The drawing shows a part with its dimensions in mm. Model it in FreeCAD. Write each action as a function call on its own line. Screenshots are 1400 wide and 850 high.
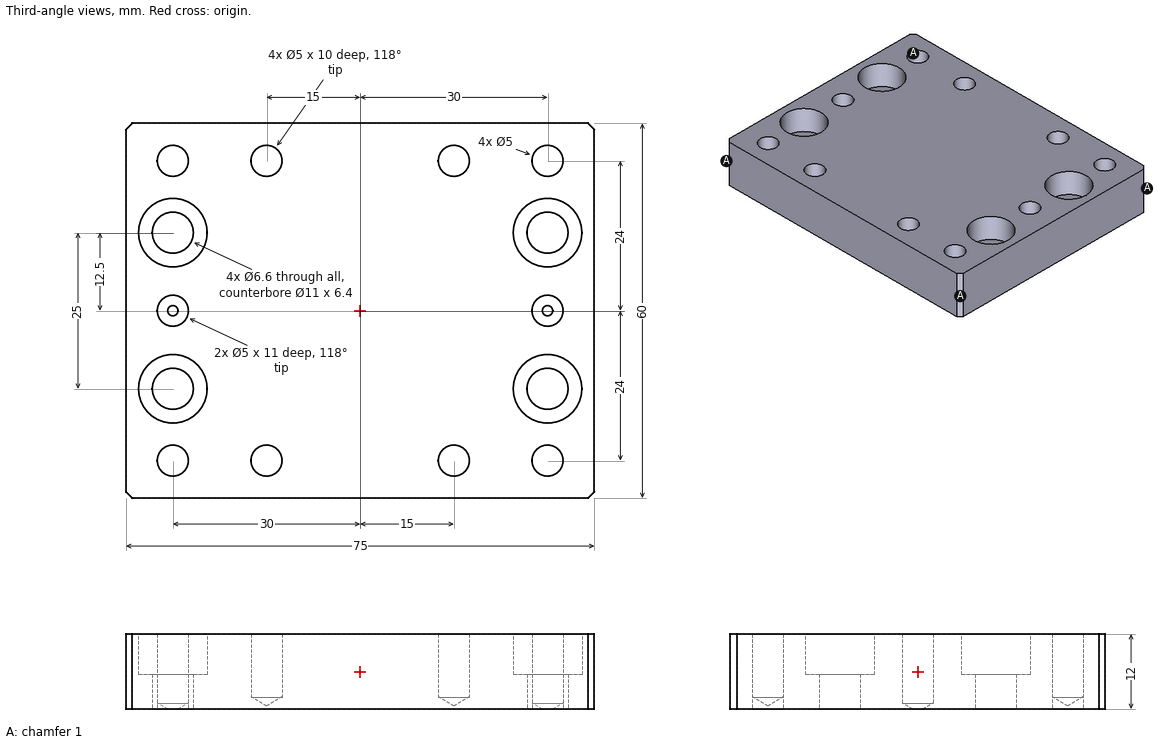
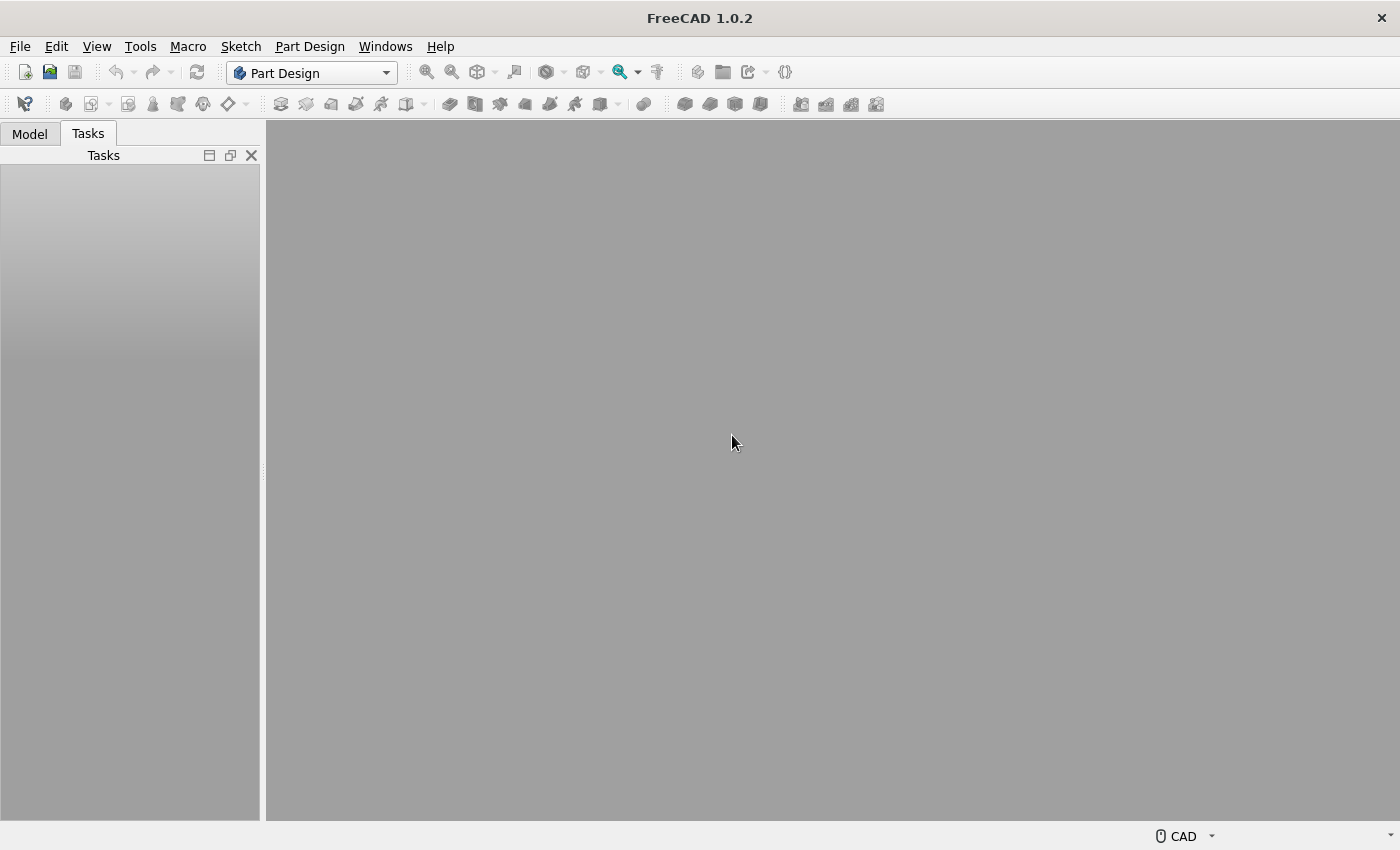
key(ctrl+n)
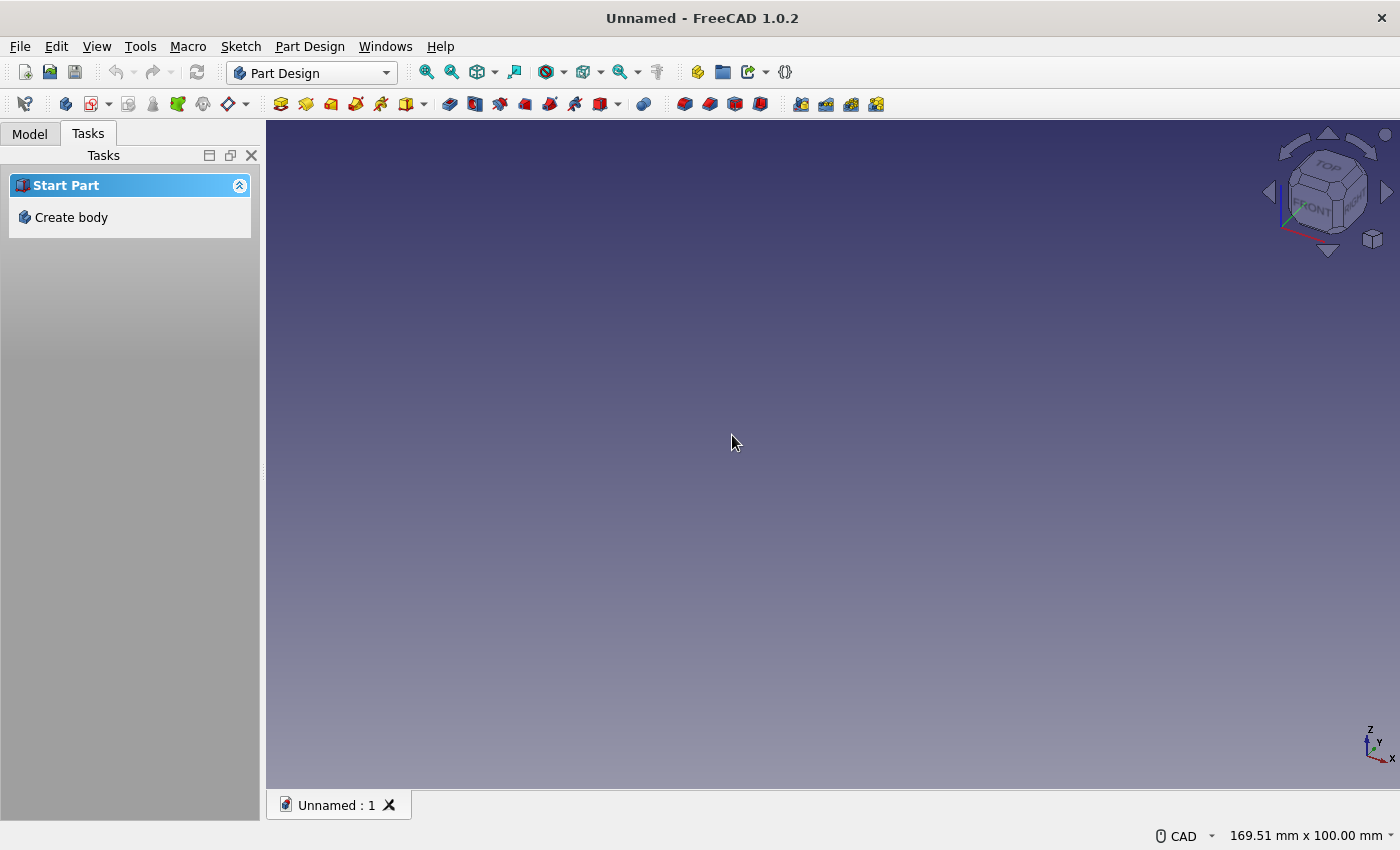
click(90, 104)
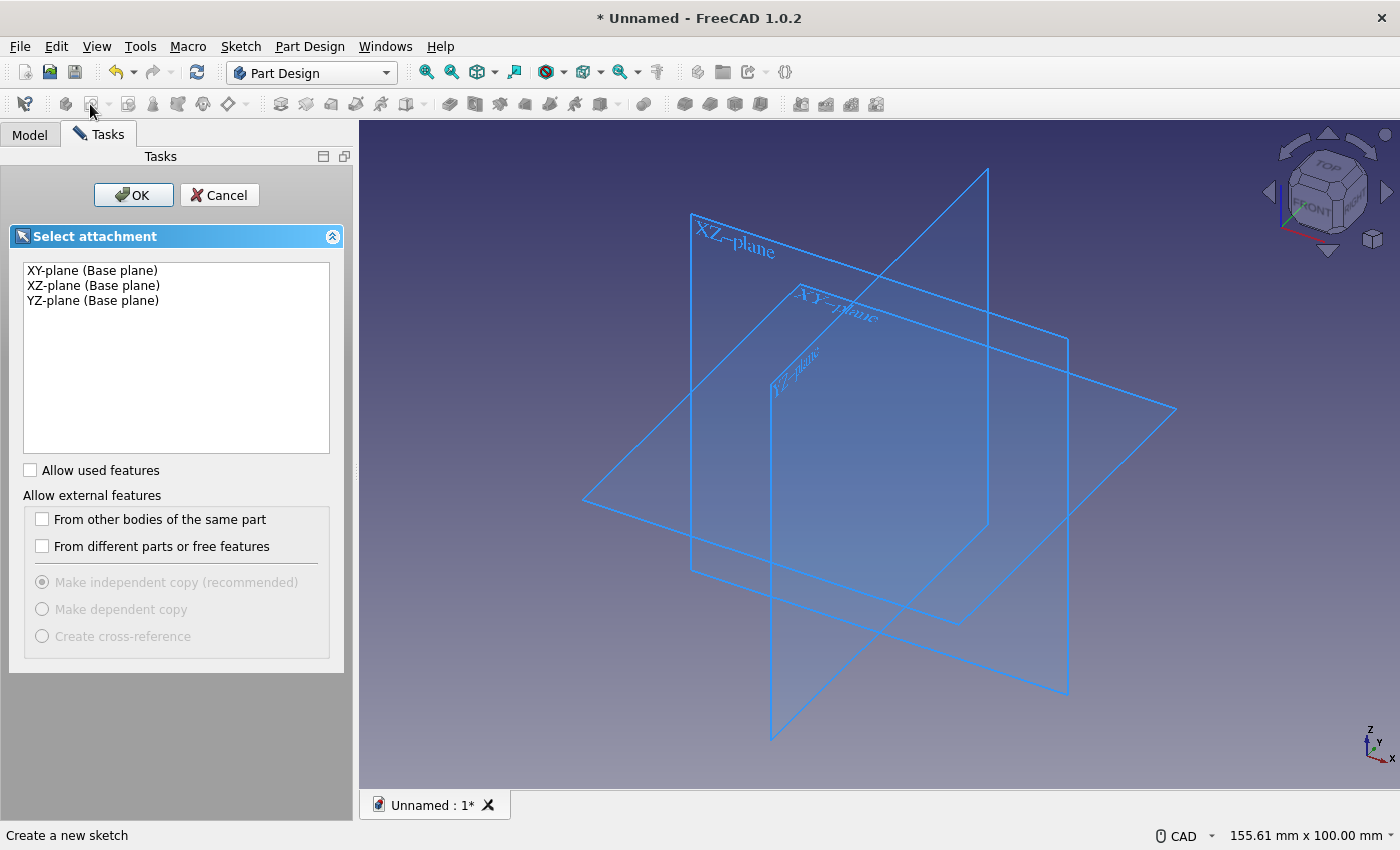
click(84, 270)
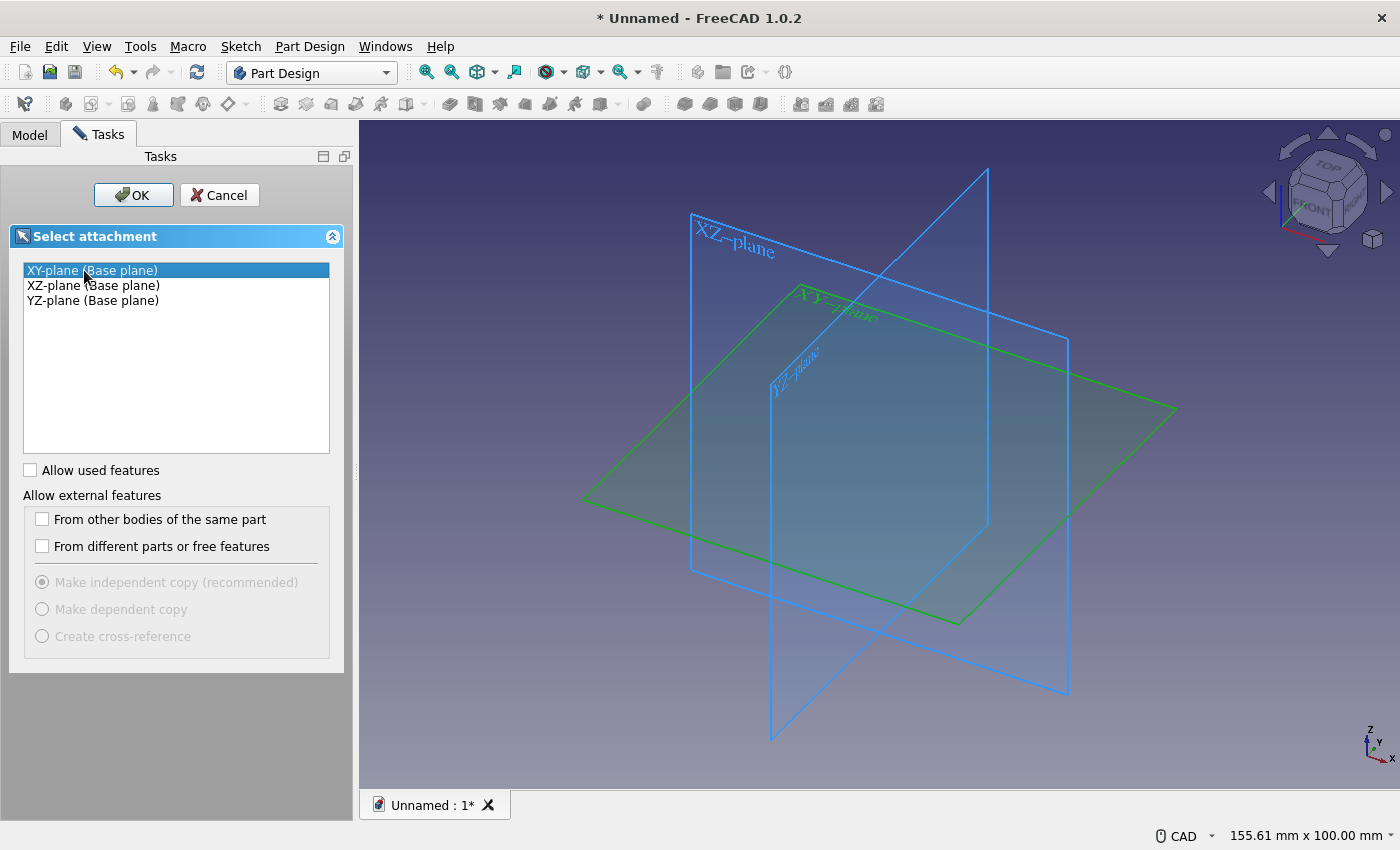
click(134, 195)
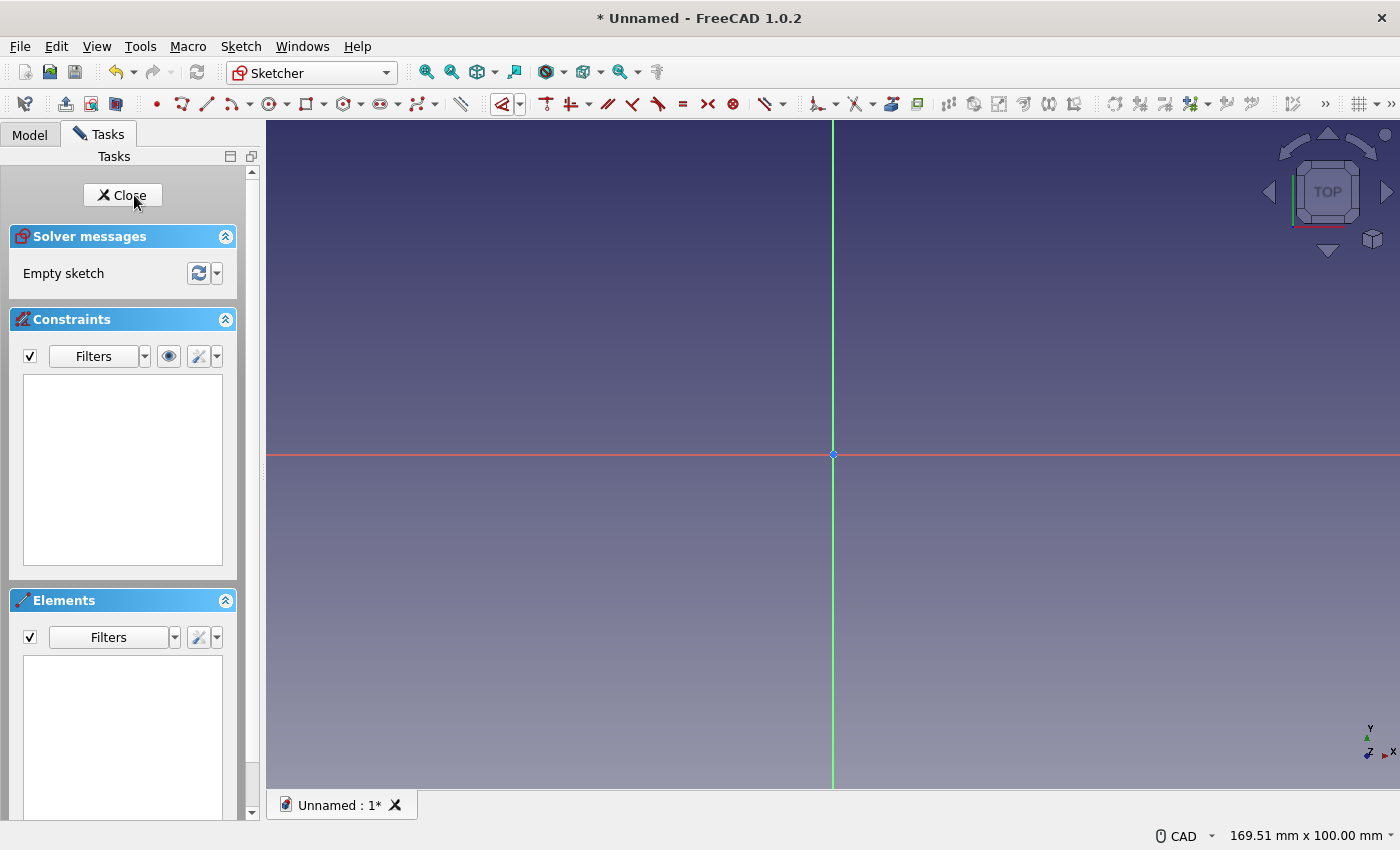
key(g)
key(v)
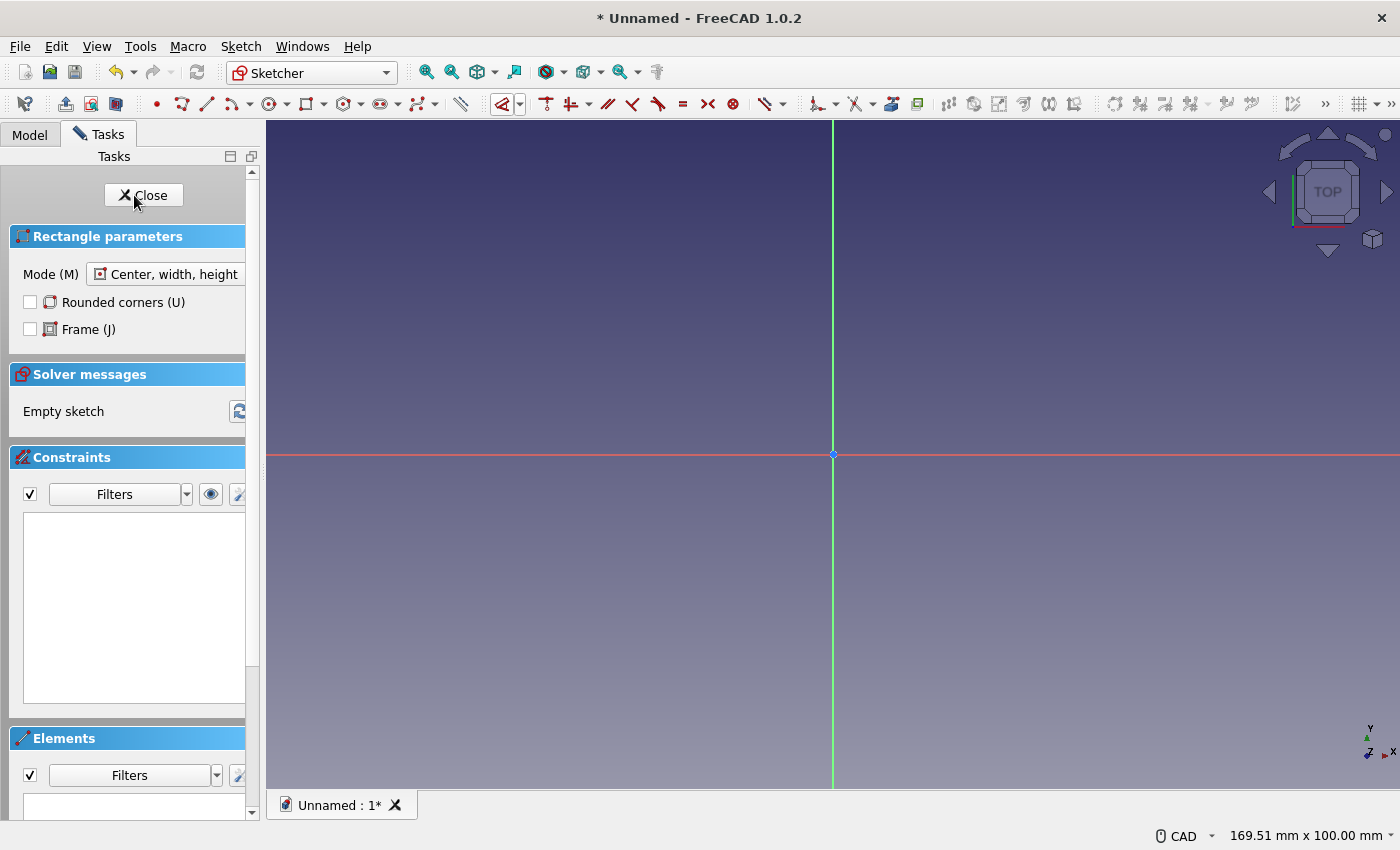
click(833, 454)
click(1084, 254)
key(Escape)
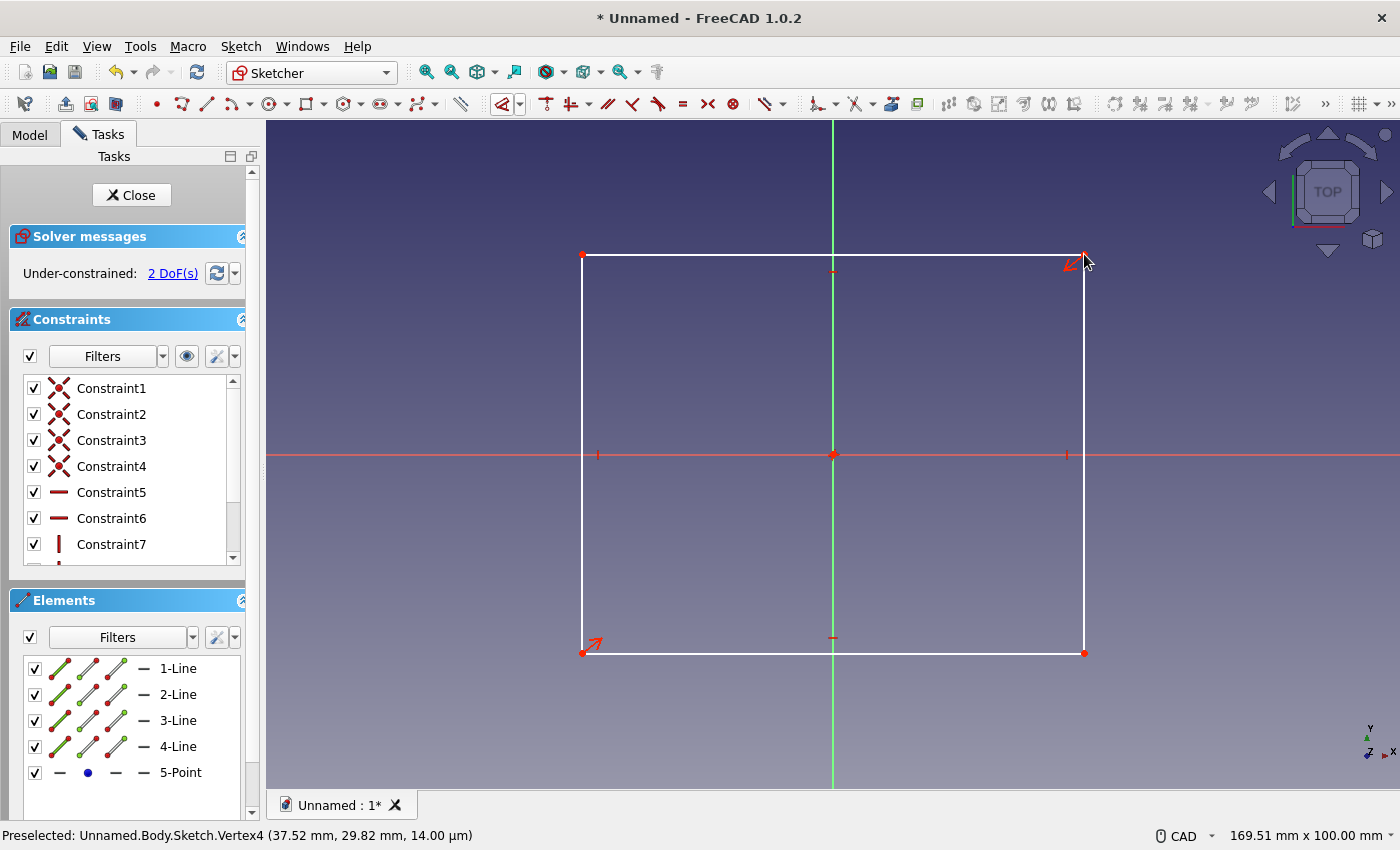
click(502, 104)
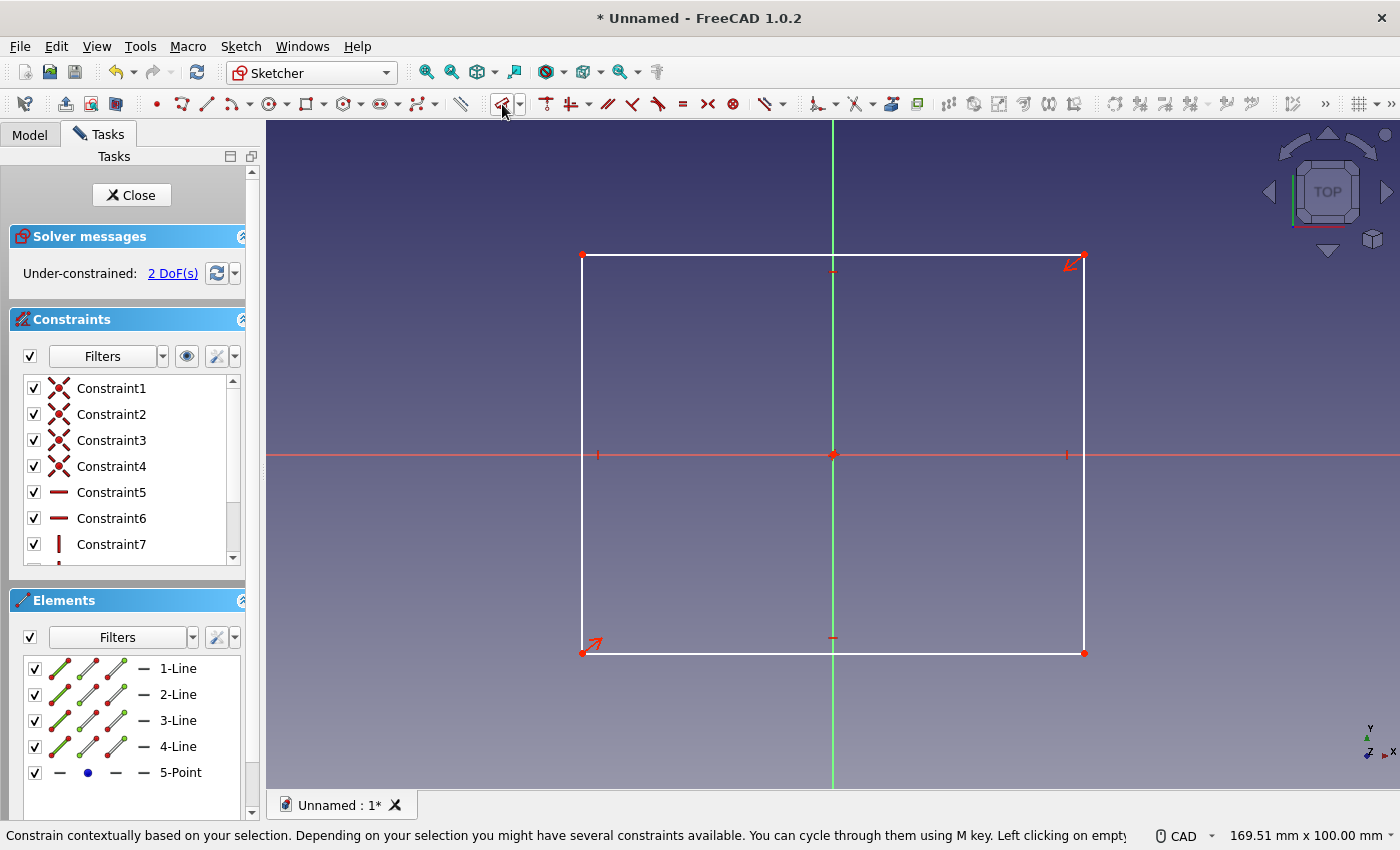
click(733, 654)
click(718, 688)